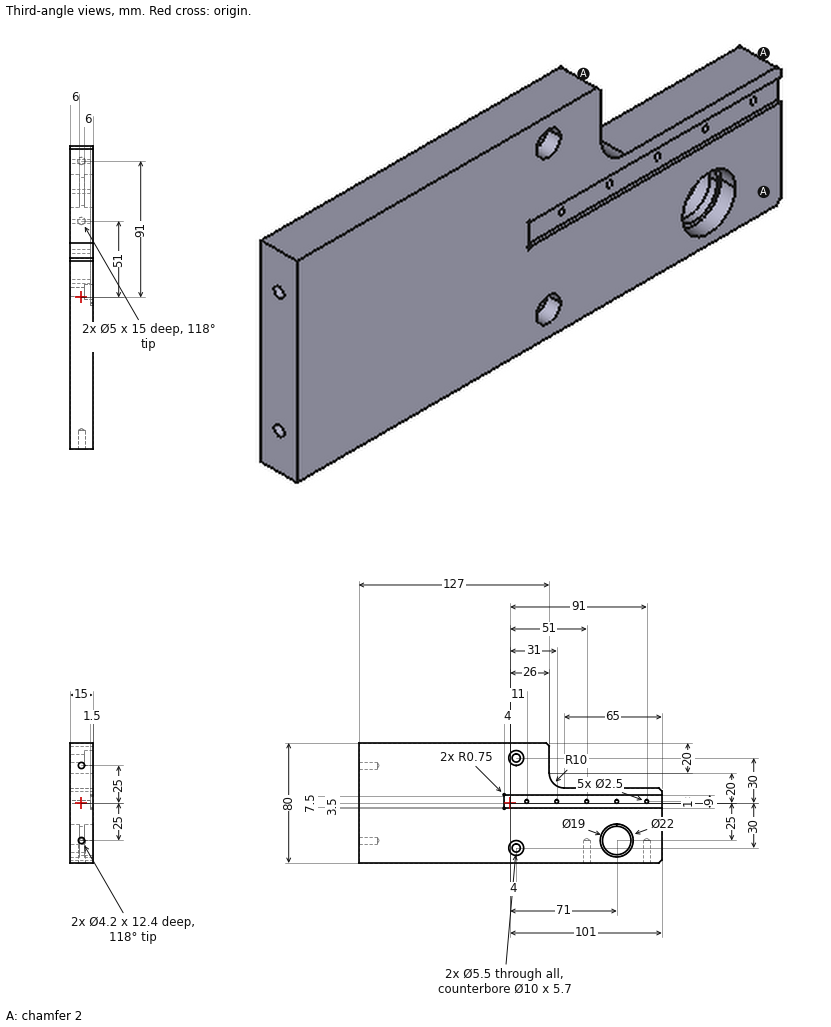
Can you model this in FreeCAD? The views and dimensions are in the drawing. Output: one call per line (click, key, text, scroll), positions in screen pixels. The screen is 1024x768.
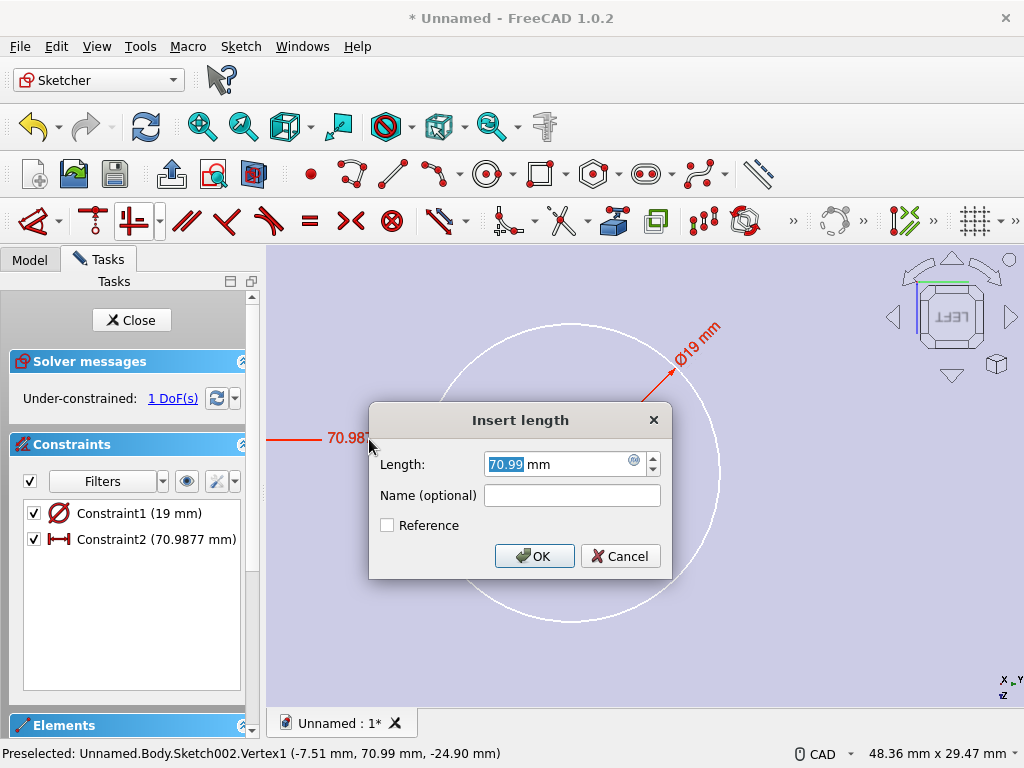
text(71)
key(Return)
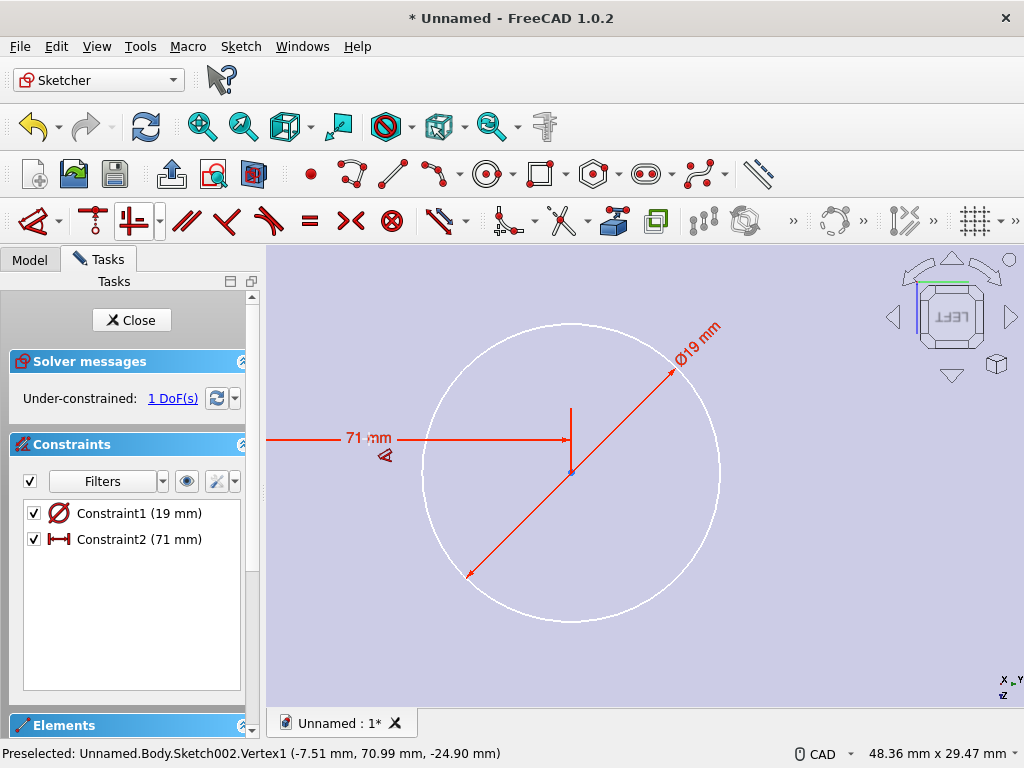
click(571, 473)
click(605, 576)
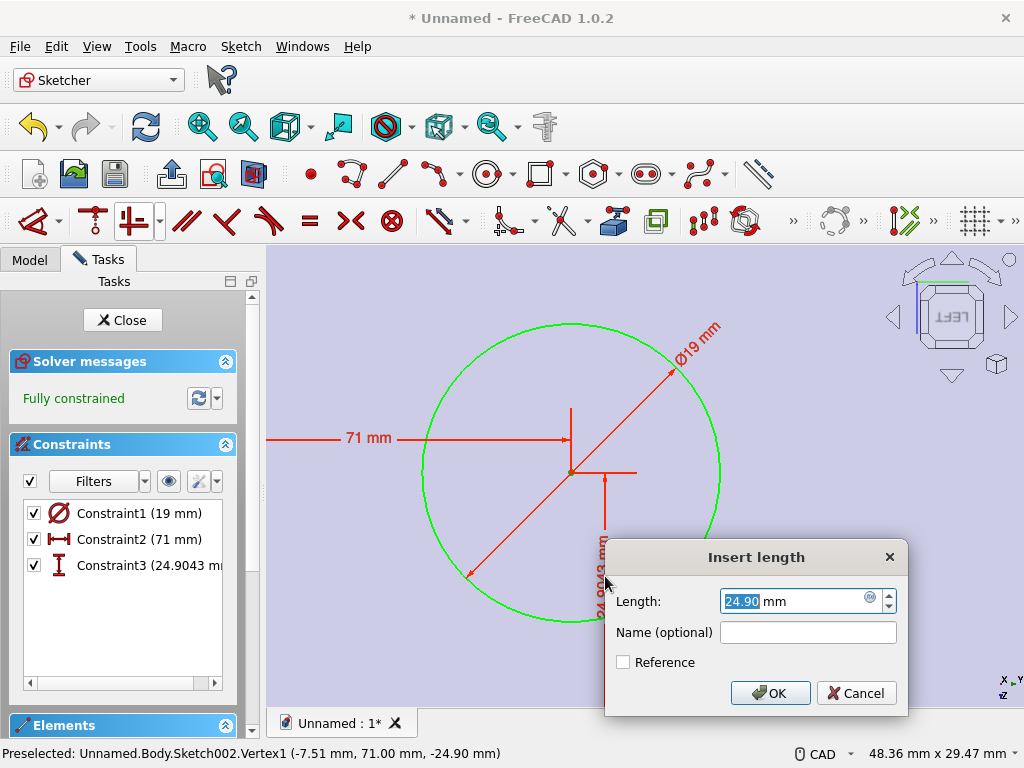
text(25)
key(Return)
key(Escape)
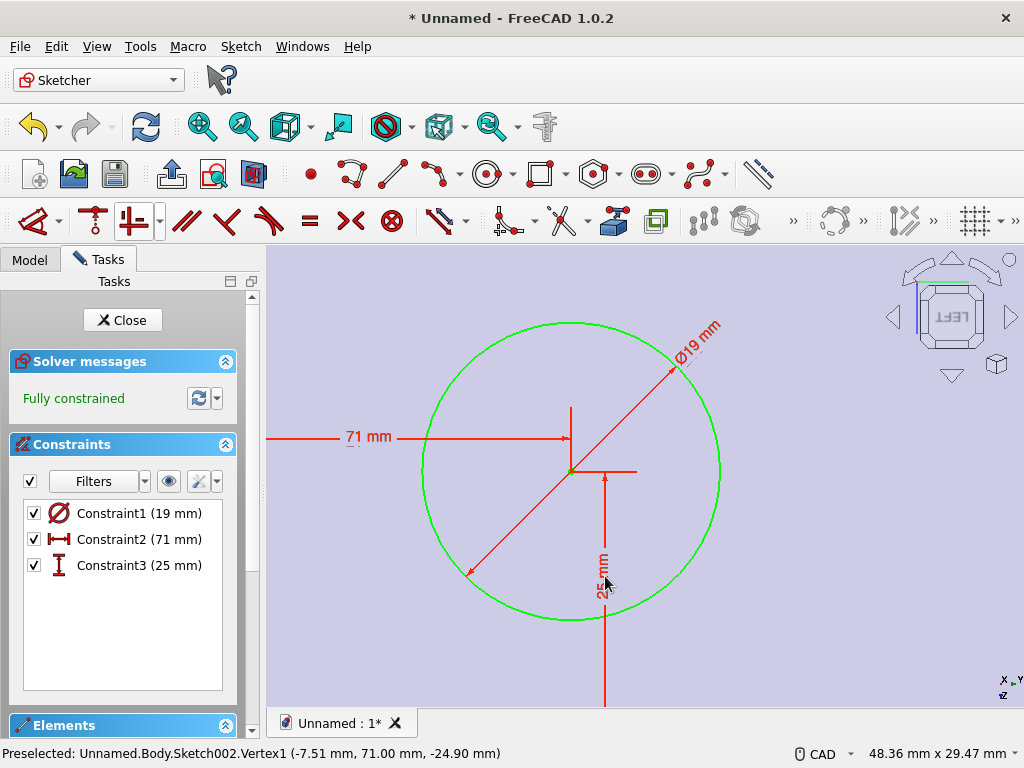
click(123, 320)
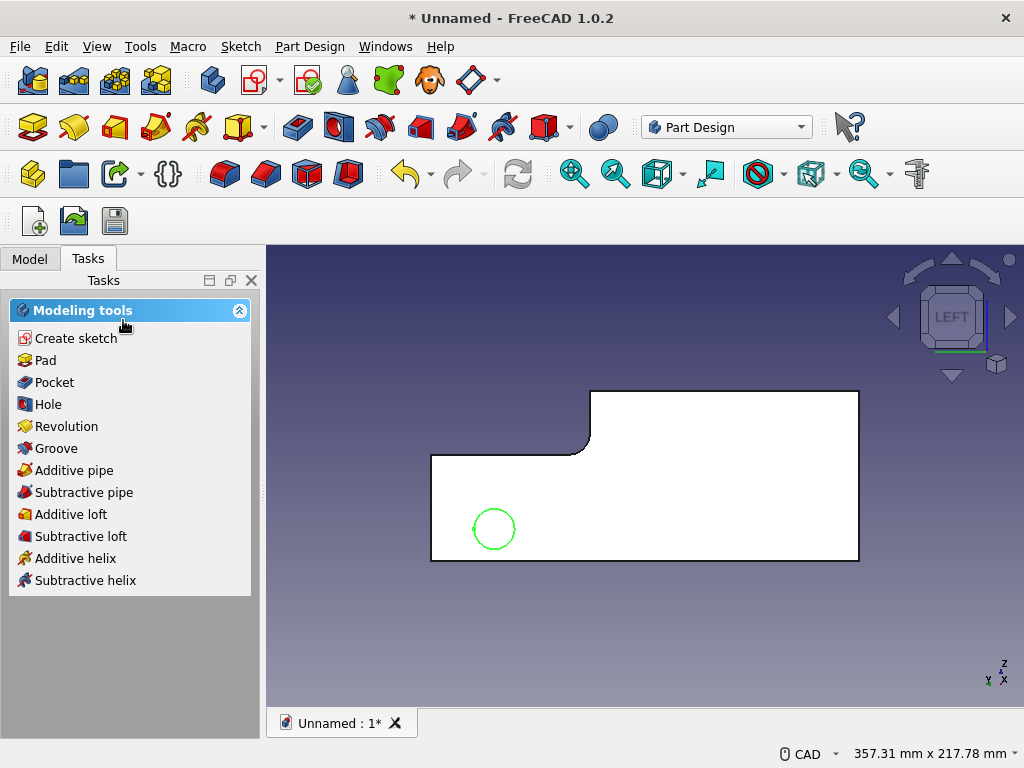
click(298, 128)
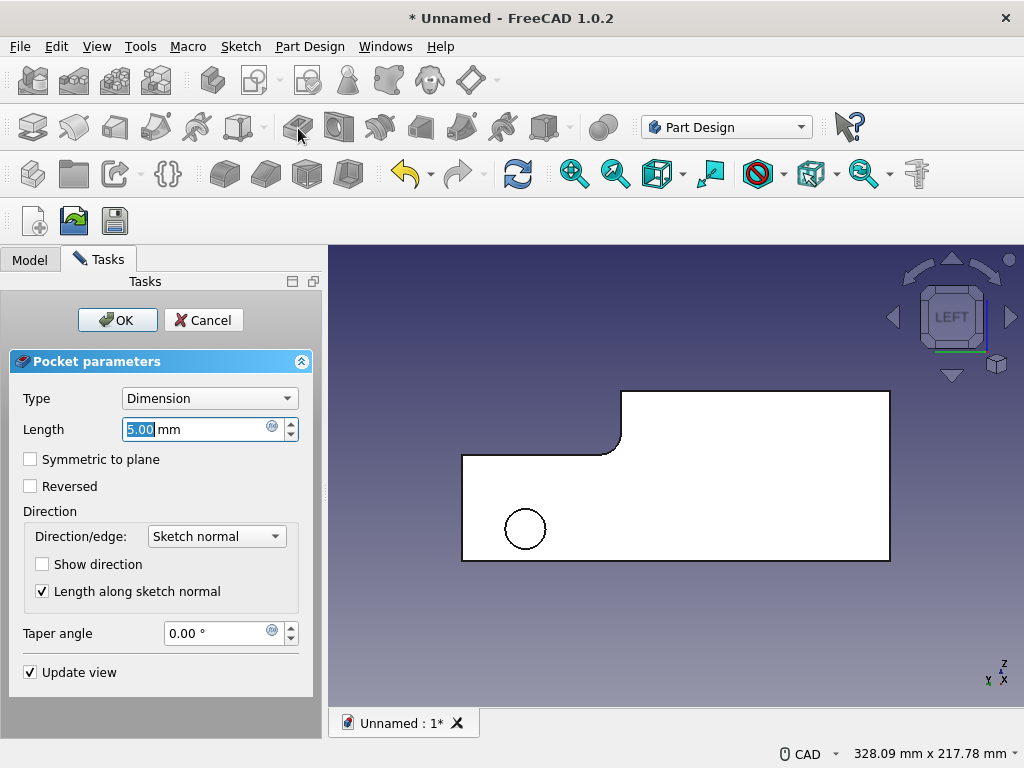
click(210, 398)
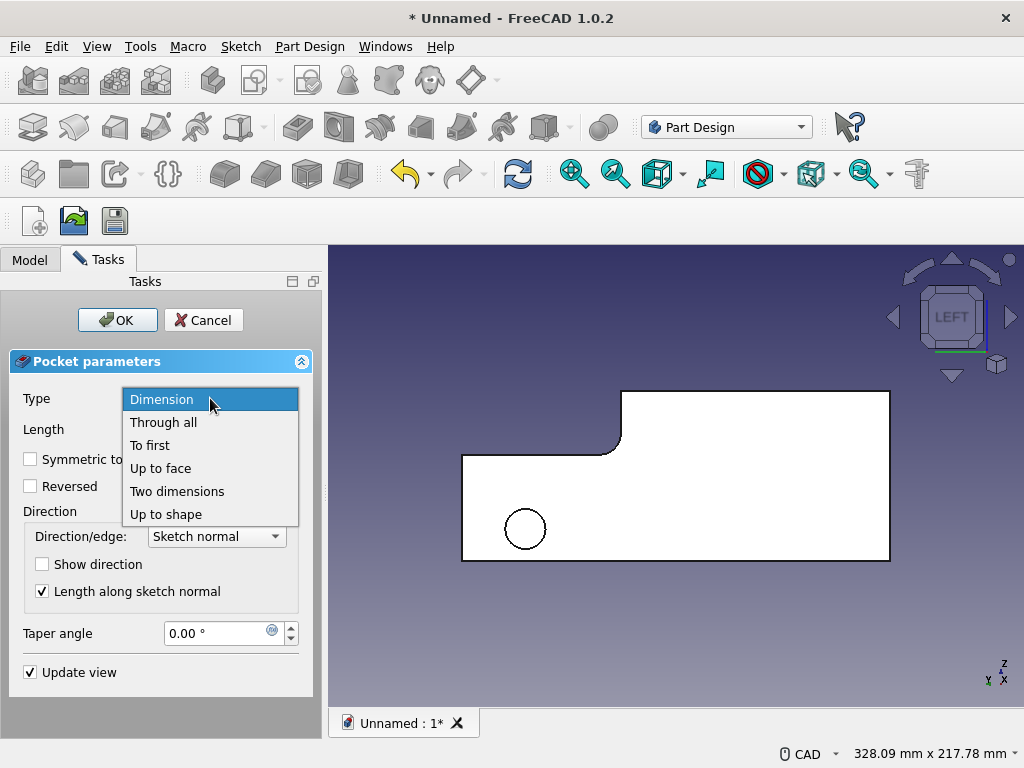
click(208, 446)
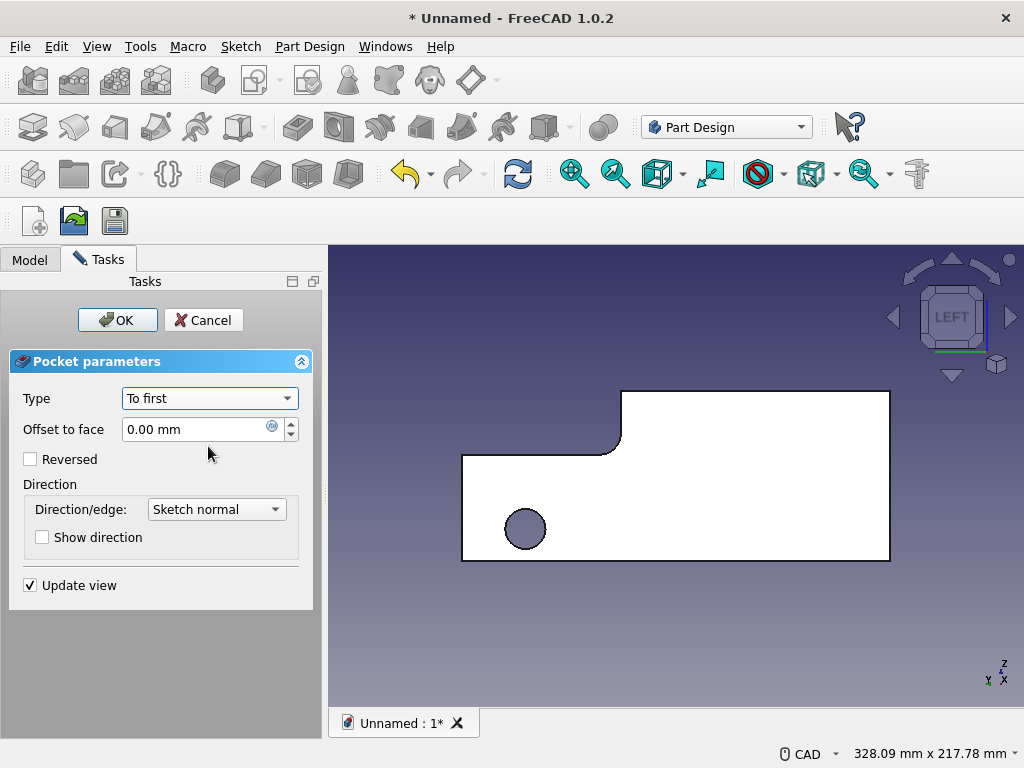
click(118, 320)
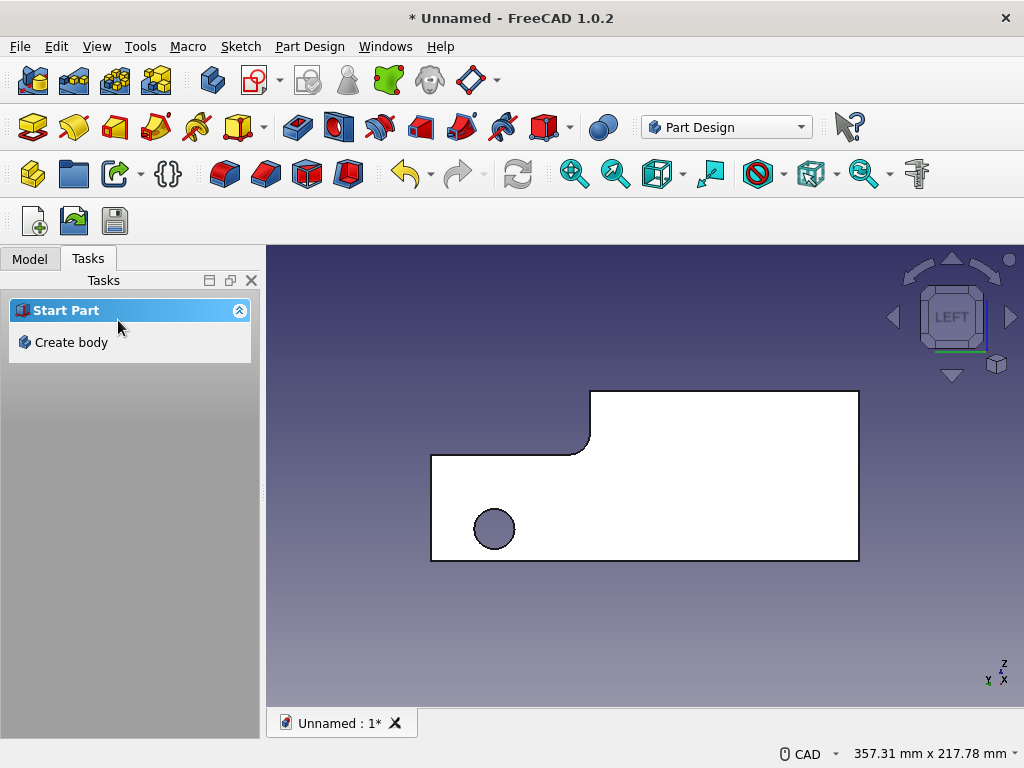
key(0)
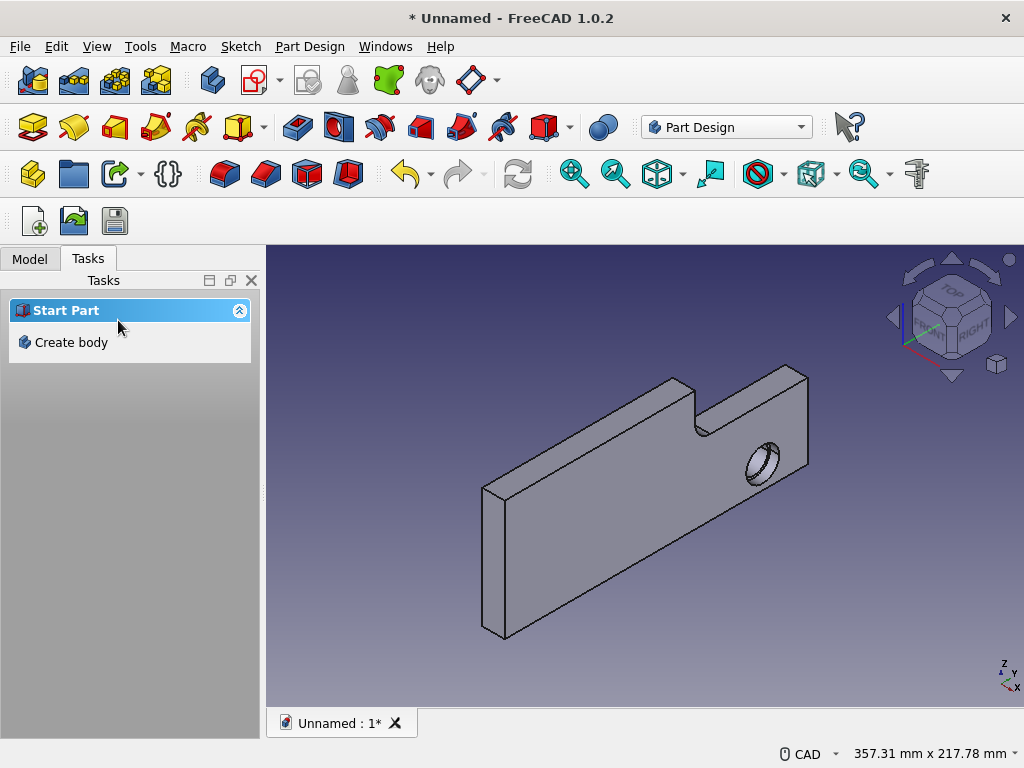
click(613, 506)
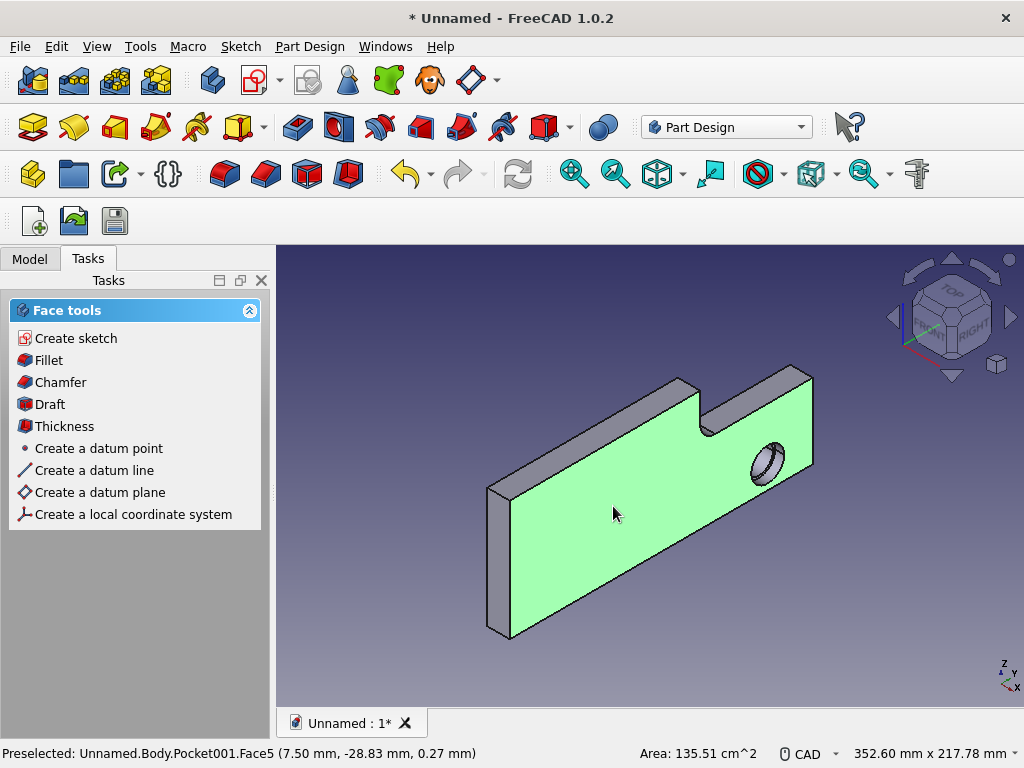
click(254, 80)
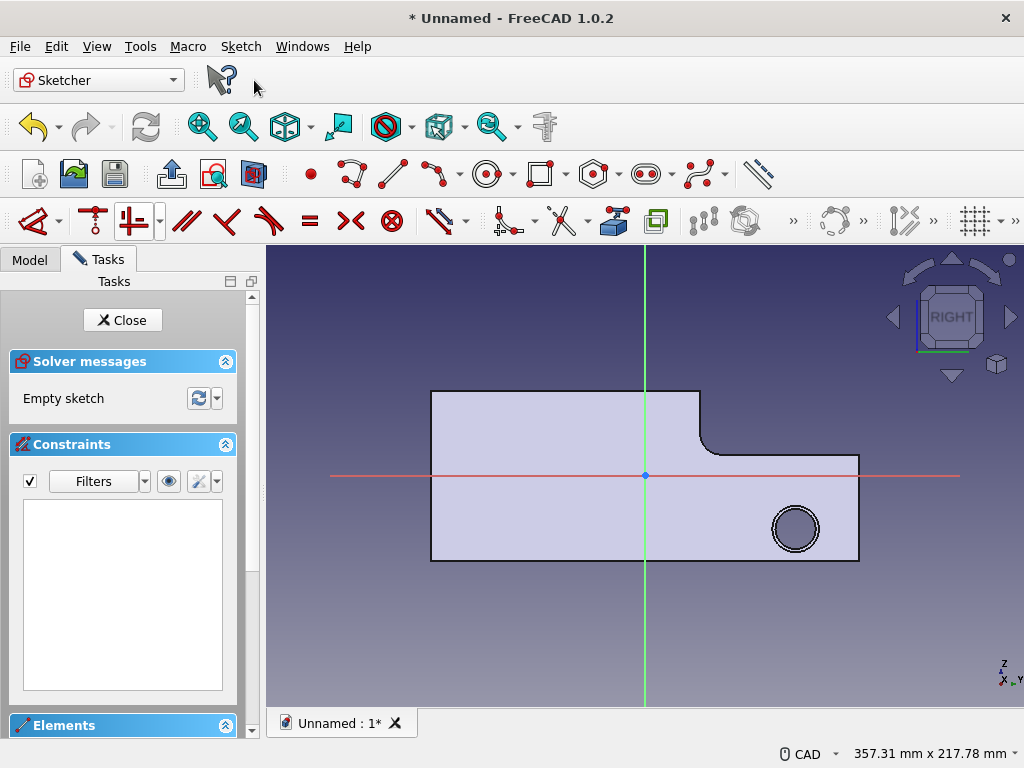
scroll(576, 476, down, 5)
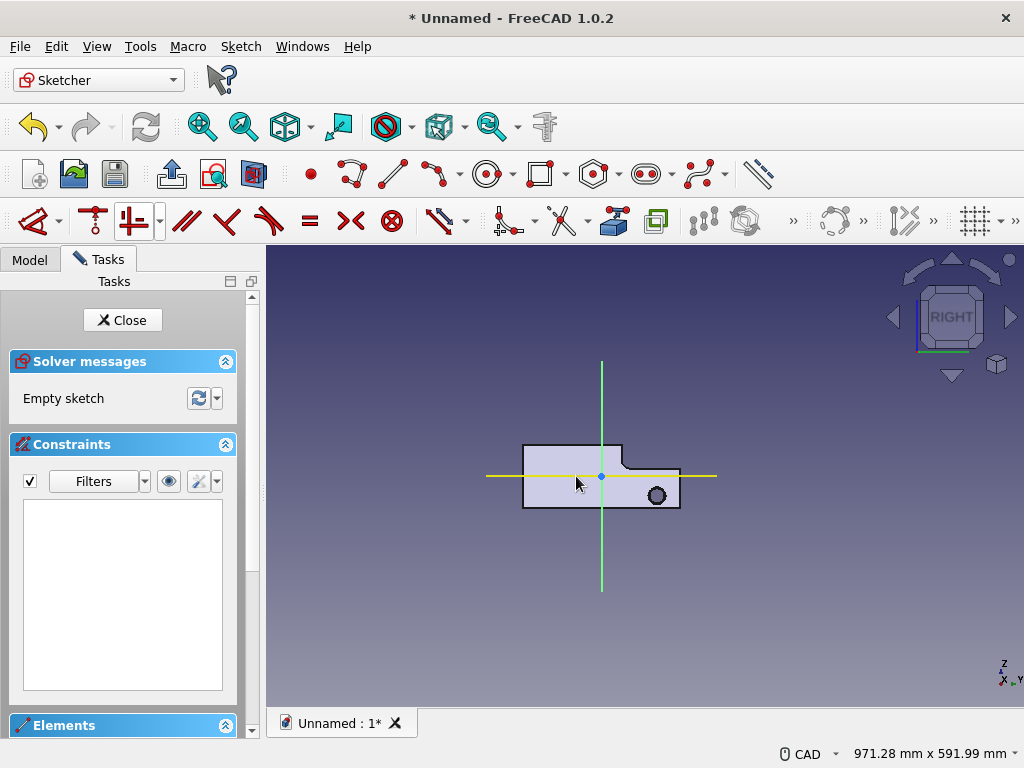
scroll(655, 475, up, 8)